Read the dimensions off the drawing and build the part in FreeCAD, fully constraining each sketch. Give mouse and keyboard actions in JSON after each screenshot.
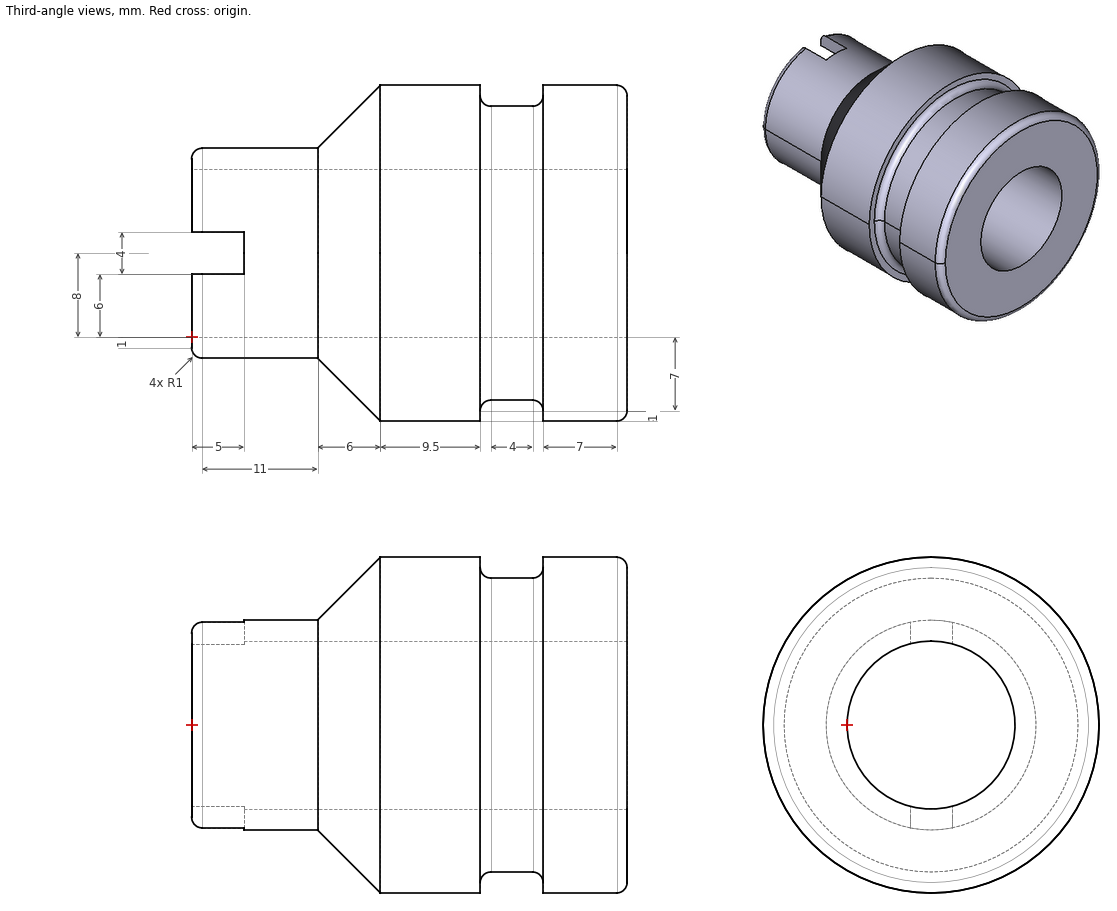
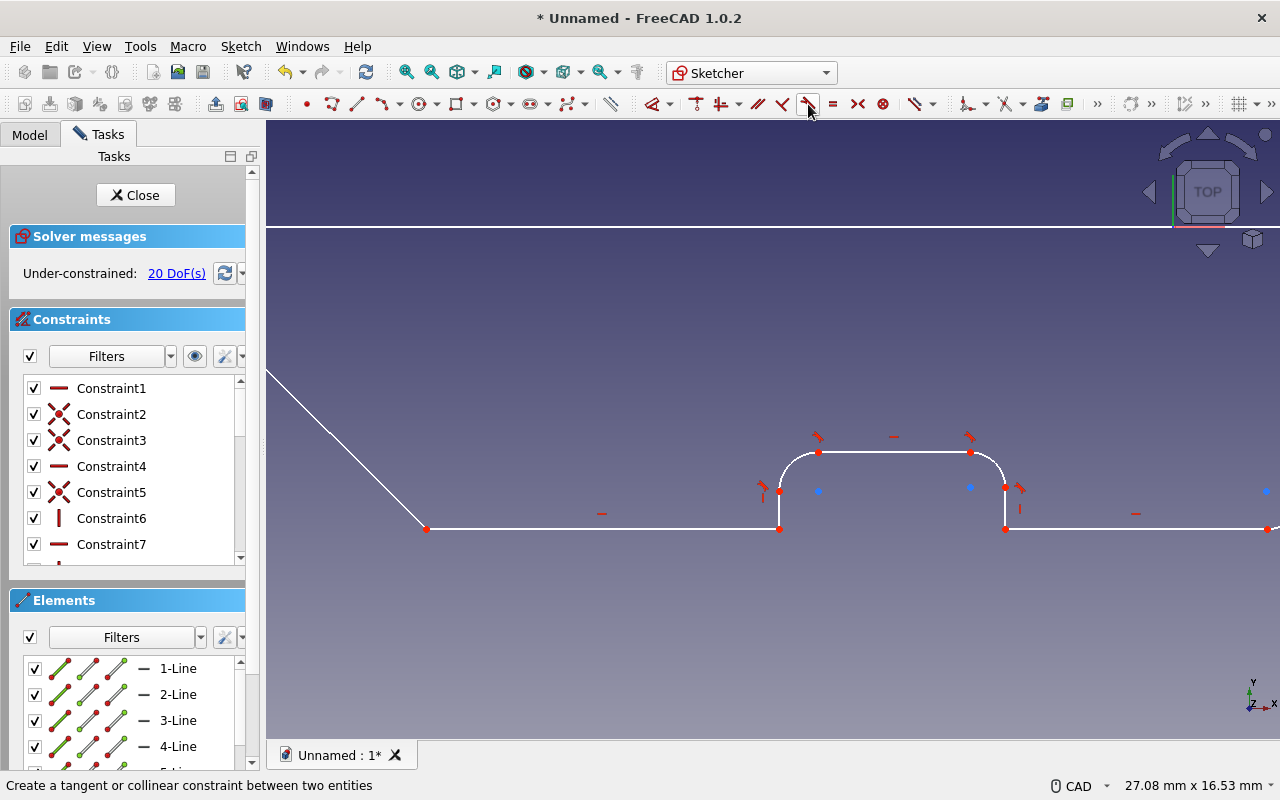
{"action": "left_click", "coordinate": [1084, 529]}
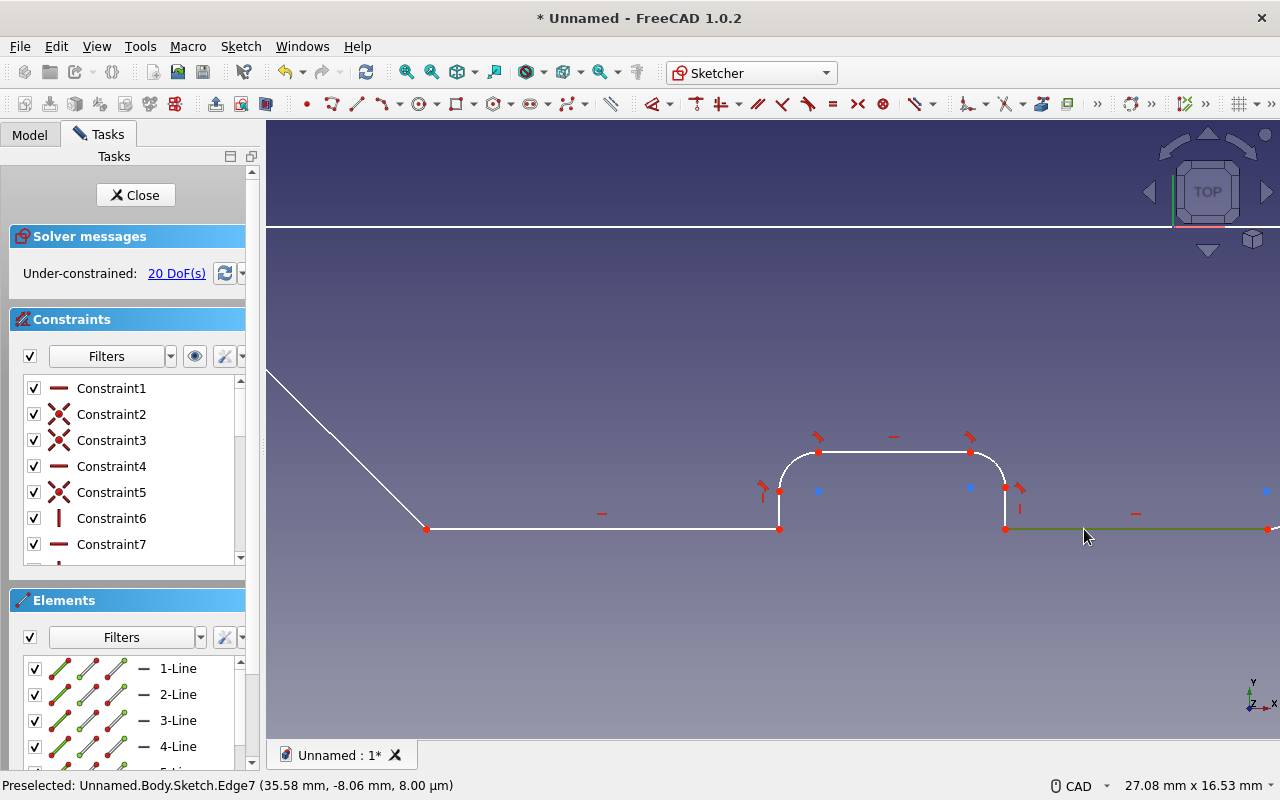
{"action": "scroll", "coordinate": [780, 517], "scroll_direction": "down", "scroll_amount": 6}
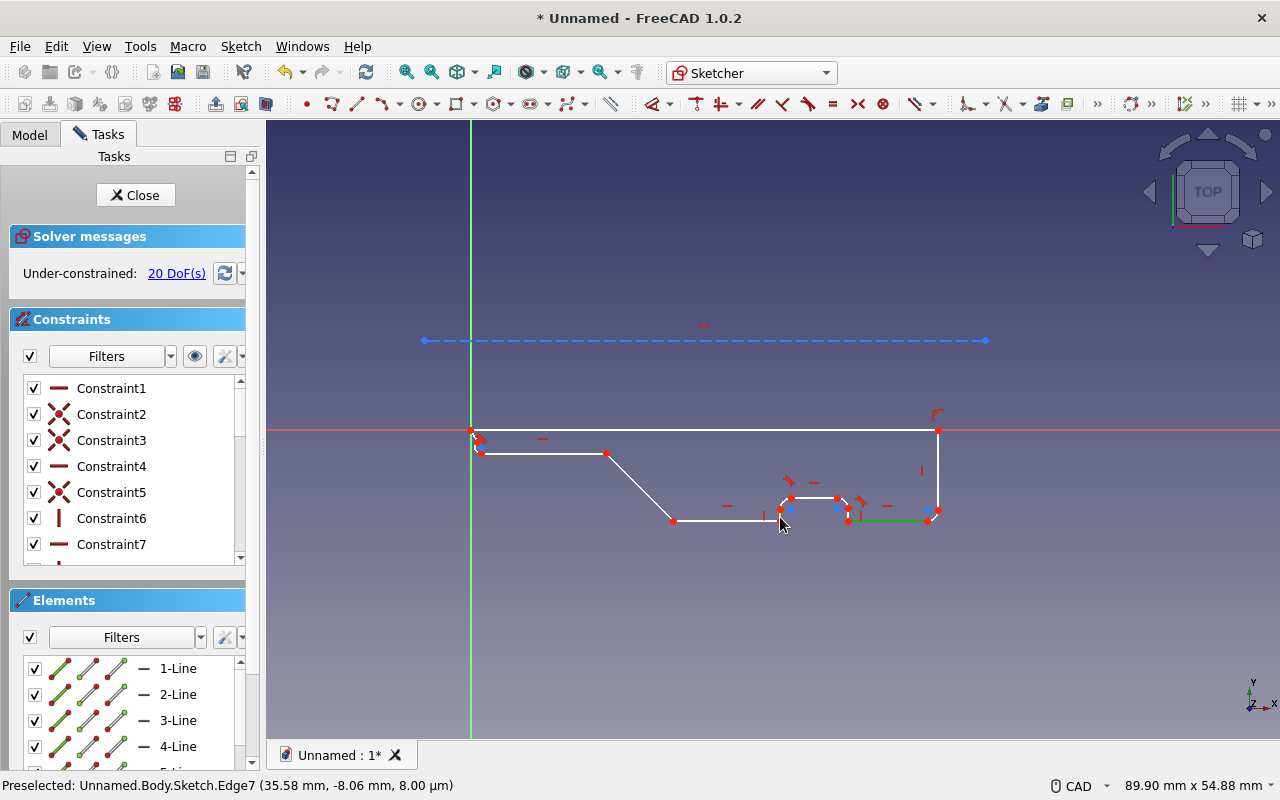
{"action": "scroll", "coordinate": [932, 520], "scroll_direction": "up", "scroll_amount": 6}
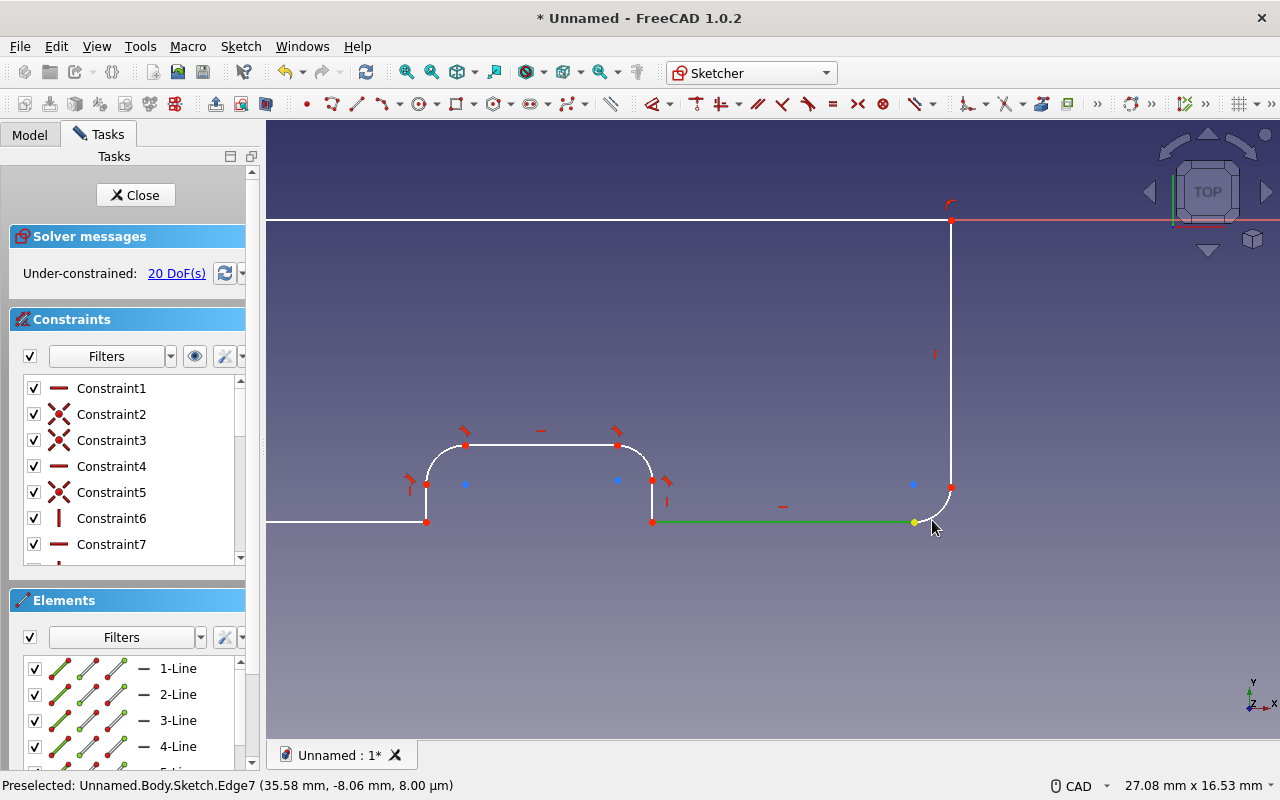
{"action": "left_click", "coordinate": [931, 518]}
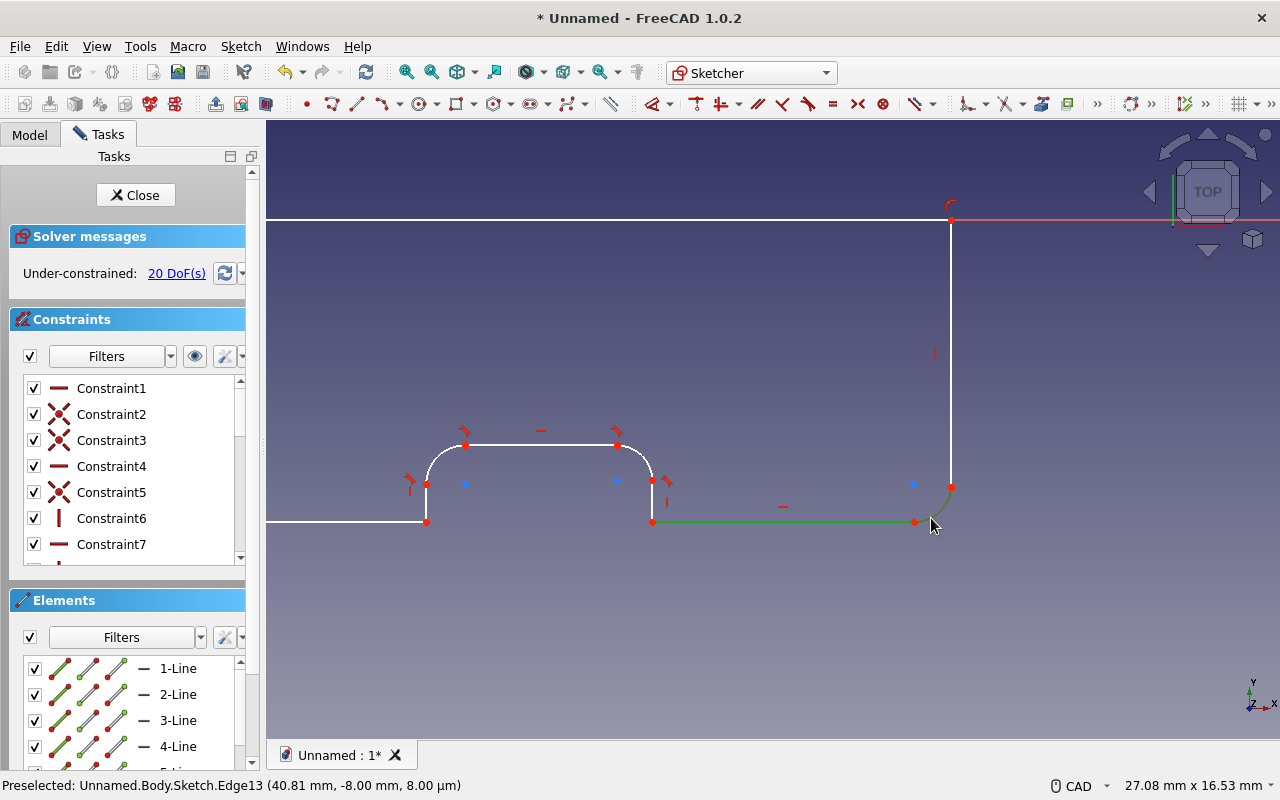
{"action": "key", "text": "t"}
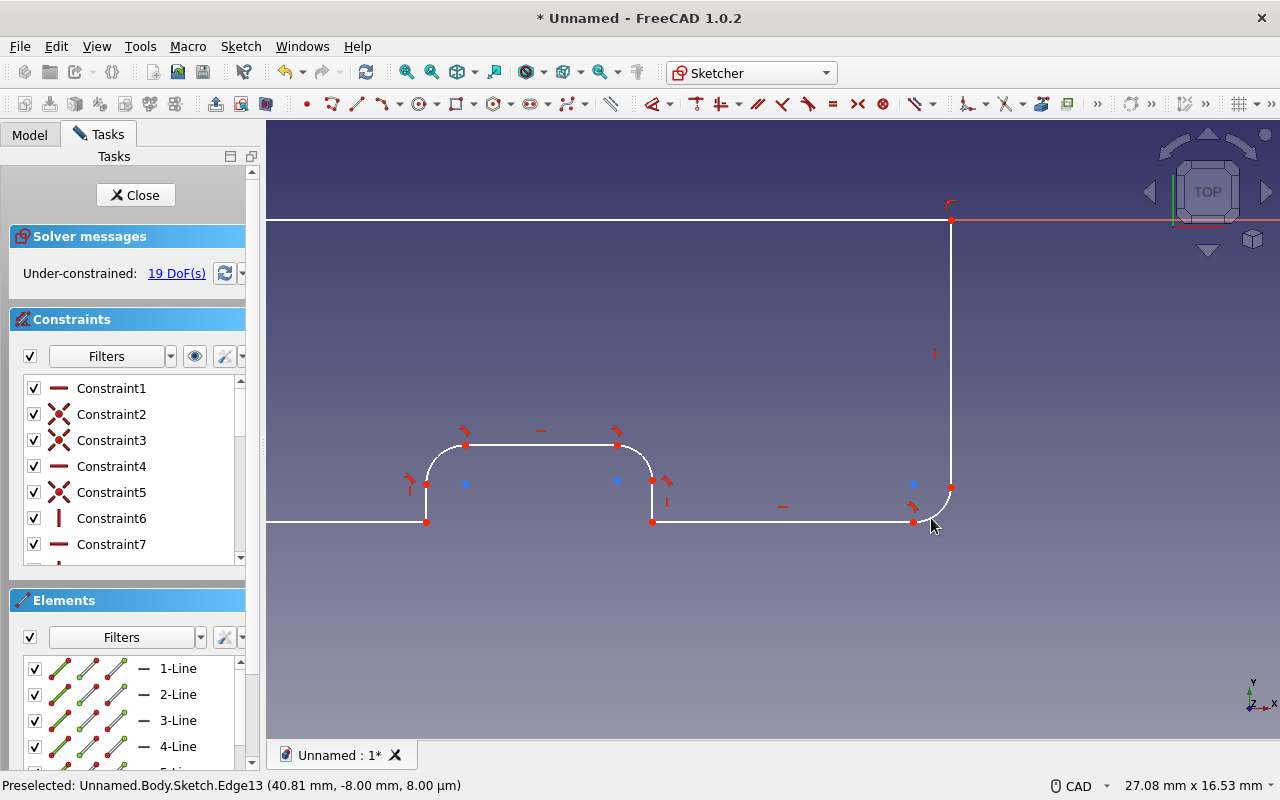
{"action": "left_click", "coordinate": [951, 407]}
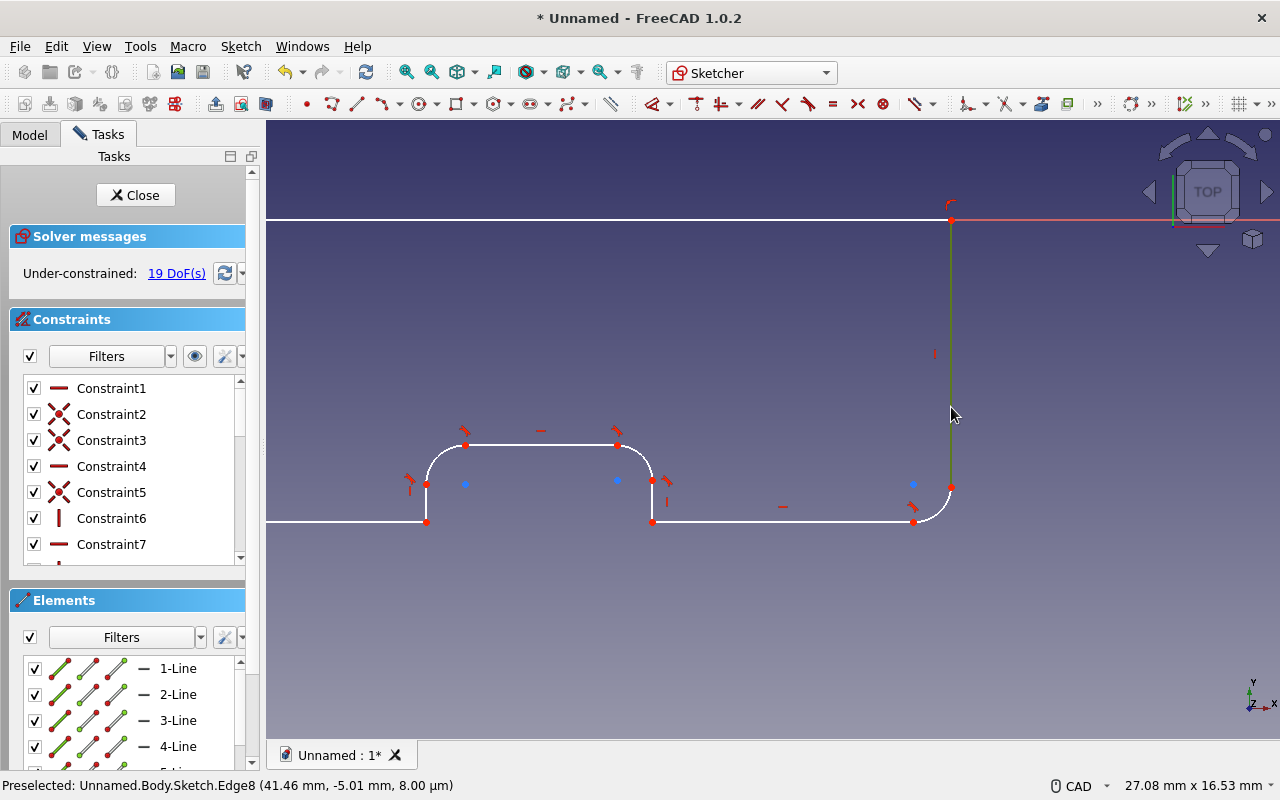
{"action": "left_click", "coordinate": [930, 518]}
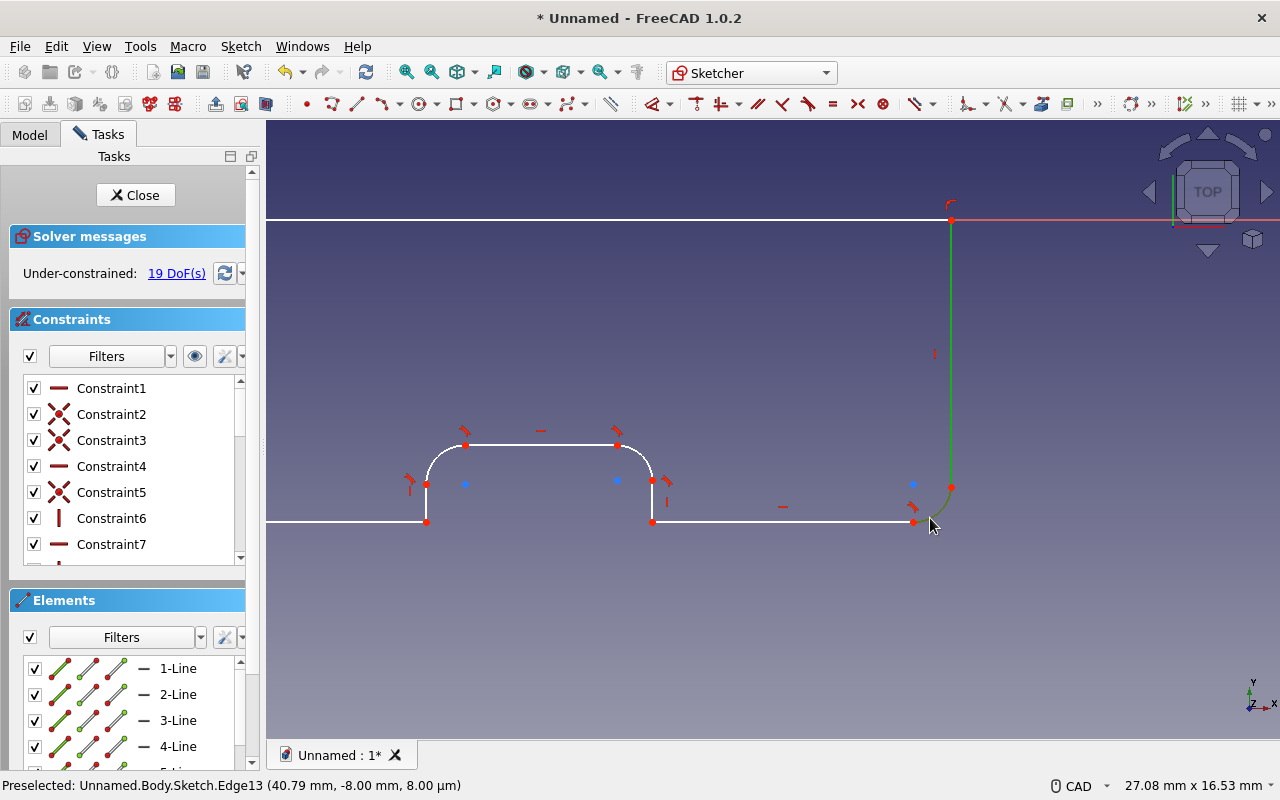
{"action": "key", "text": "t"}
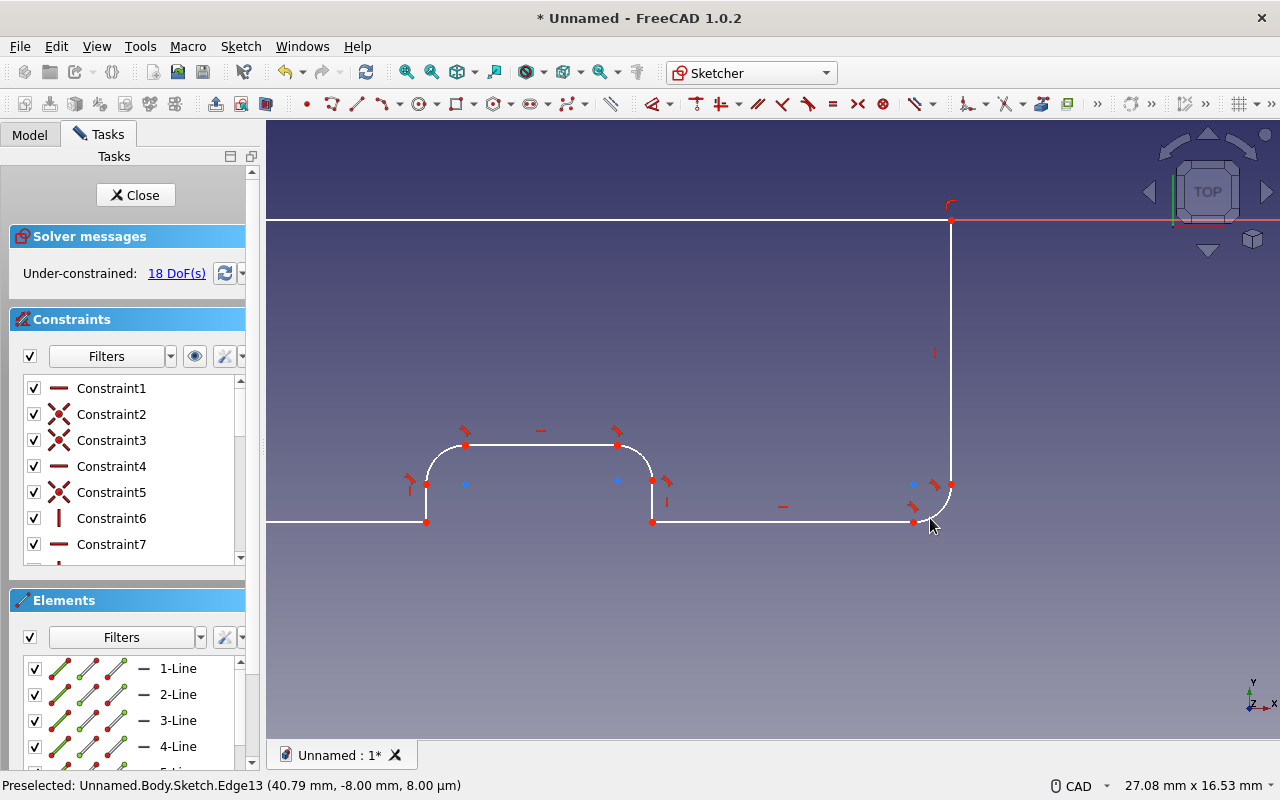
{"action": "scroll", "coordinate": [933, 520], "scroll_direction": "down", "scroll_amount": 6}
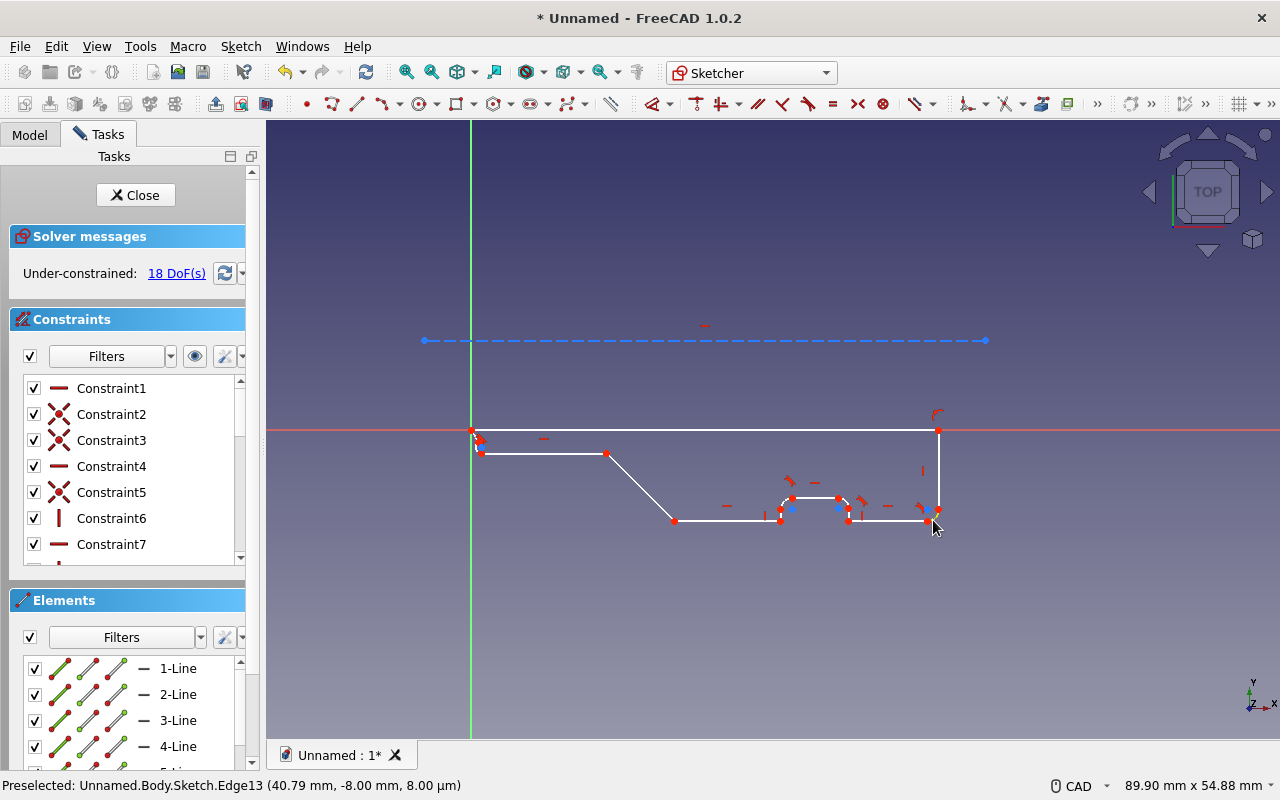
{"action": "scroll", "coordinate": [476, 439], "scroll_direction": "up", "scroll_amount": 6}